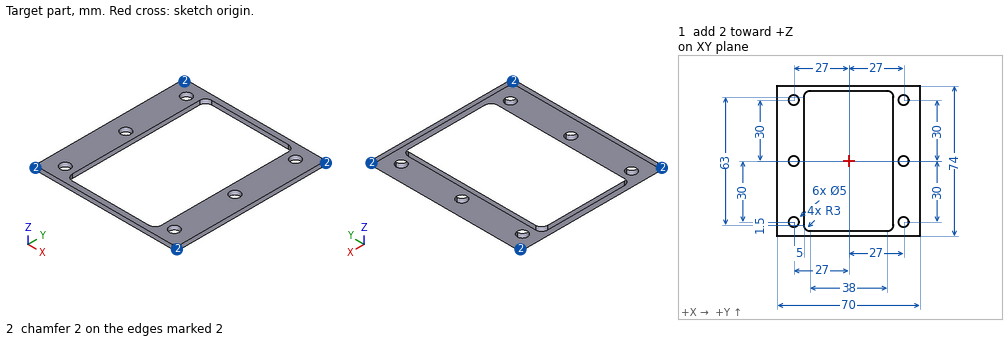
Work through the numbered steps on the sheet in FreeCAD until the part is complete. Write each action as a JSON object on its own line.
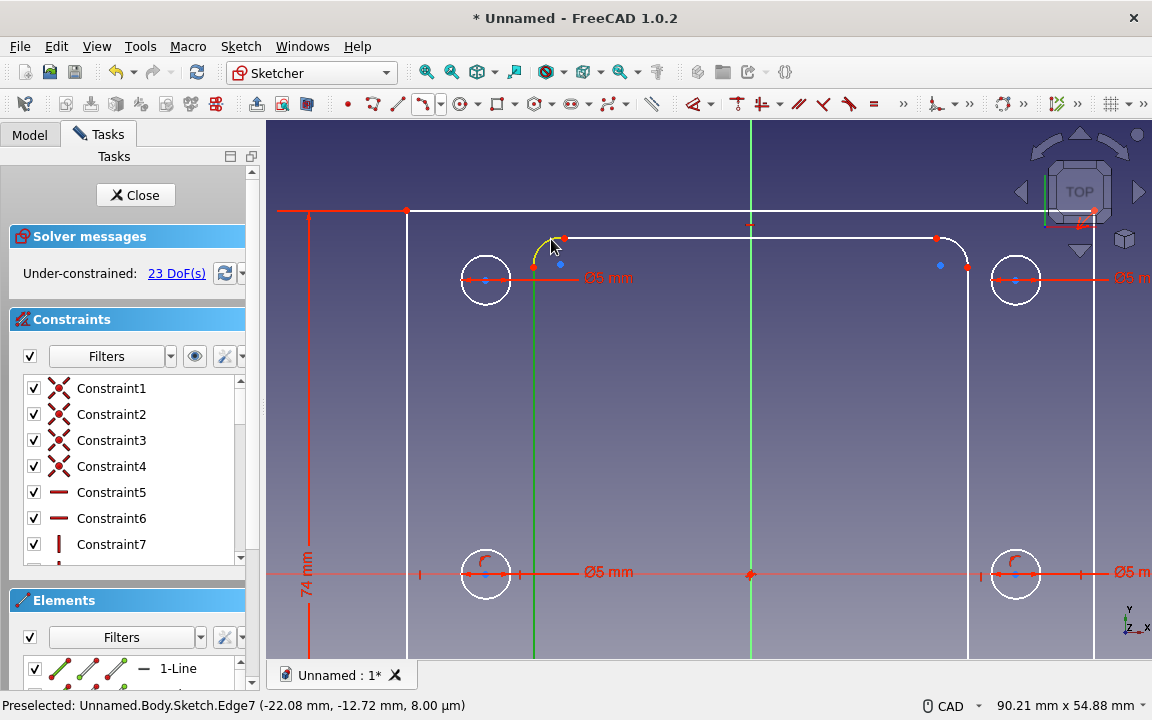
{"action": "left_click", "coordinate": [550, 240]}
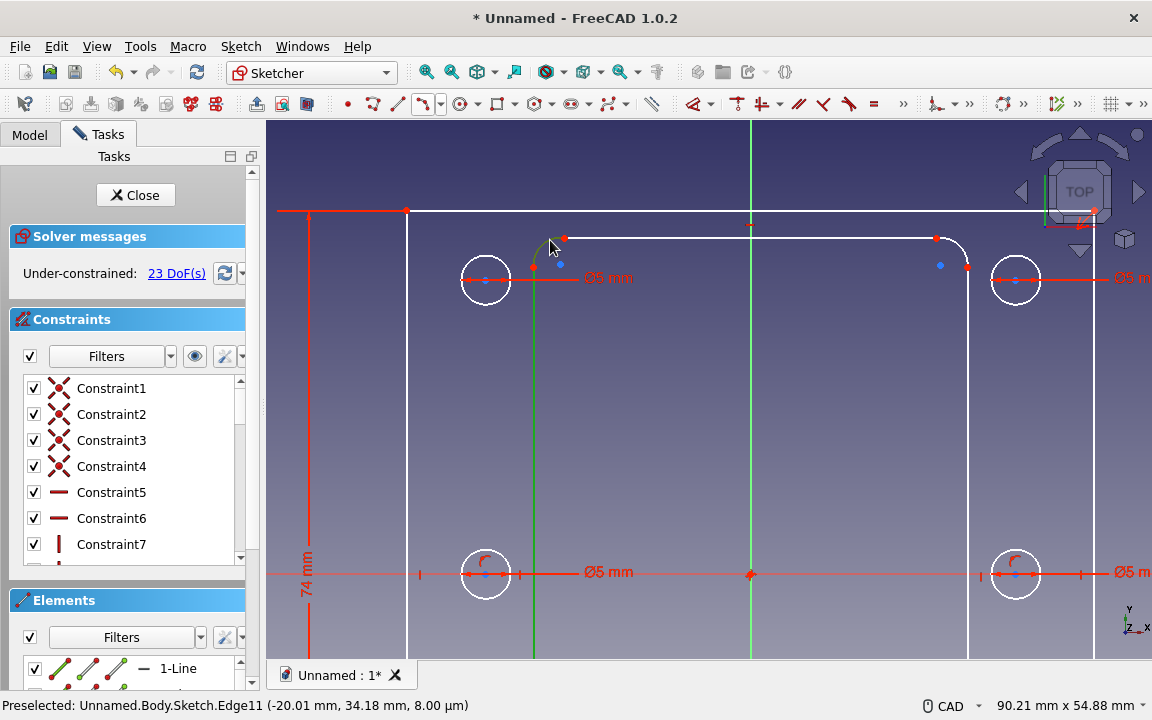
{"action": "left_click", "coordinate": [849, 104]}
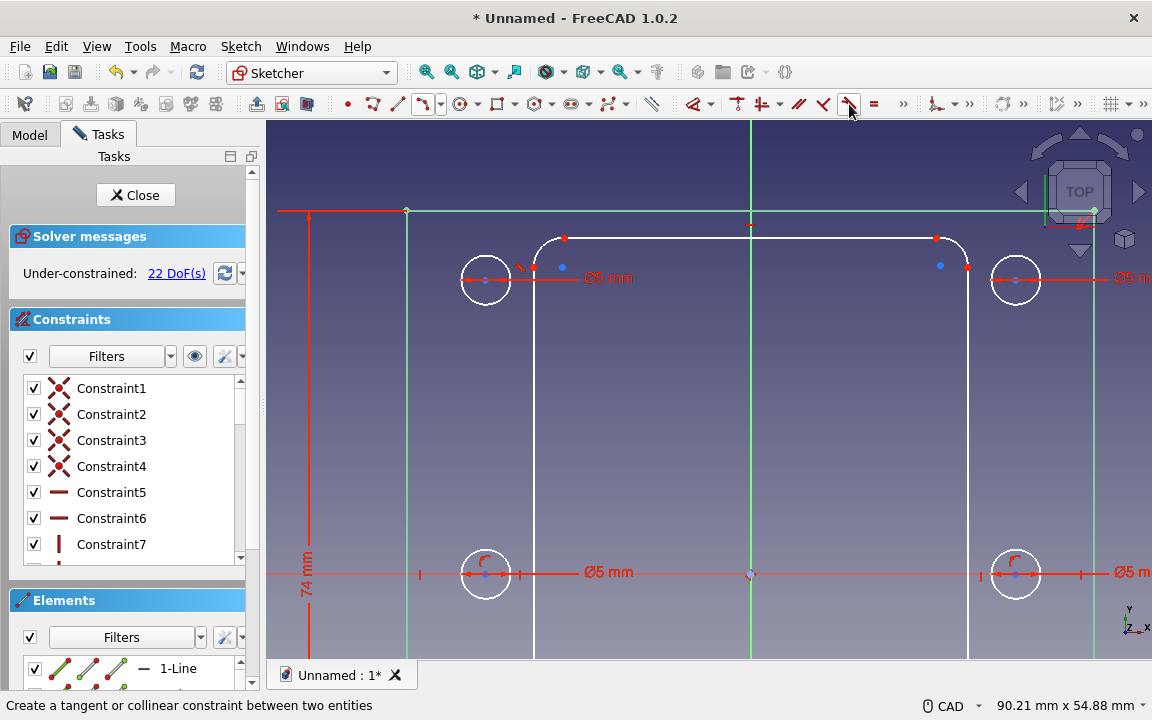
{"action": "left_click", "coordinate": [676, 238]}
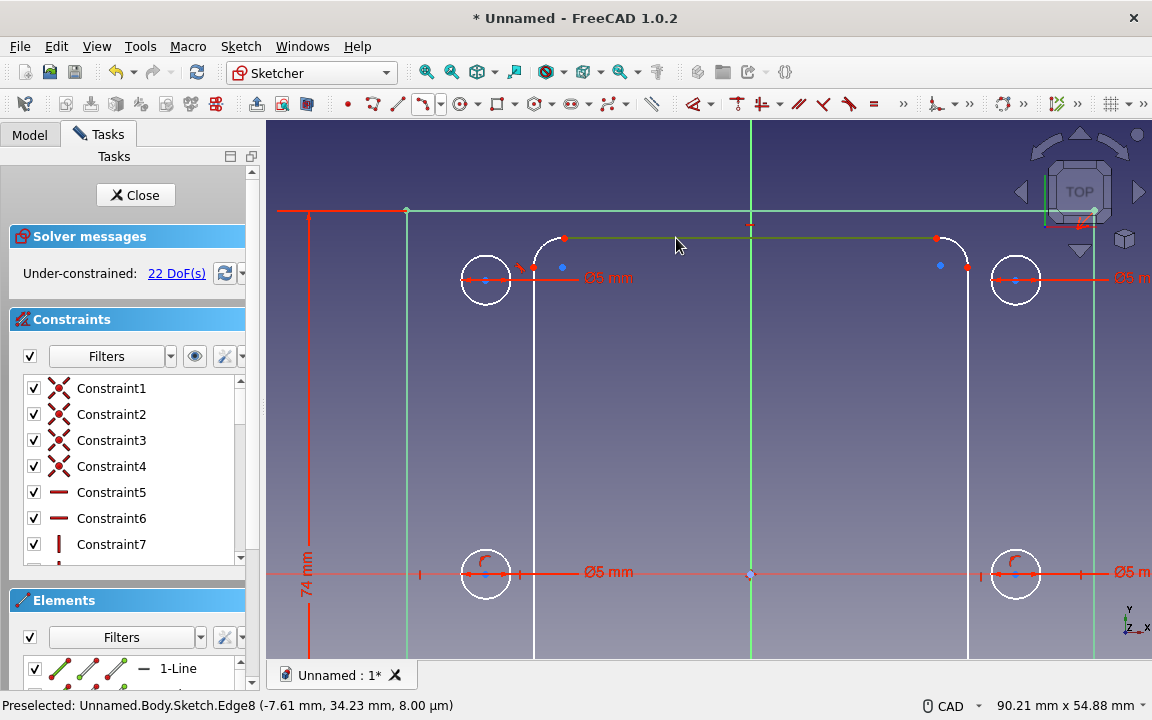
{"action": "left_click", "coordinate": [551, 241]}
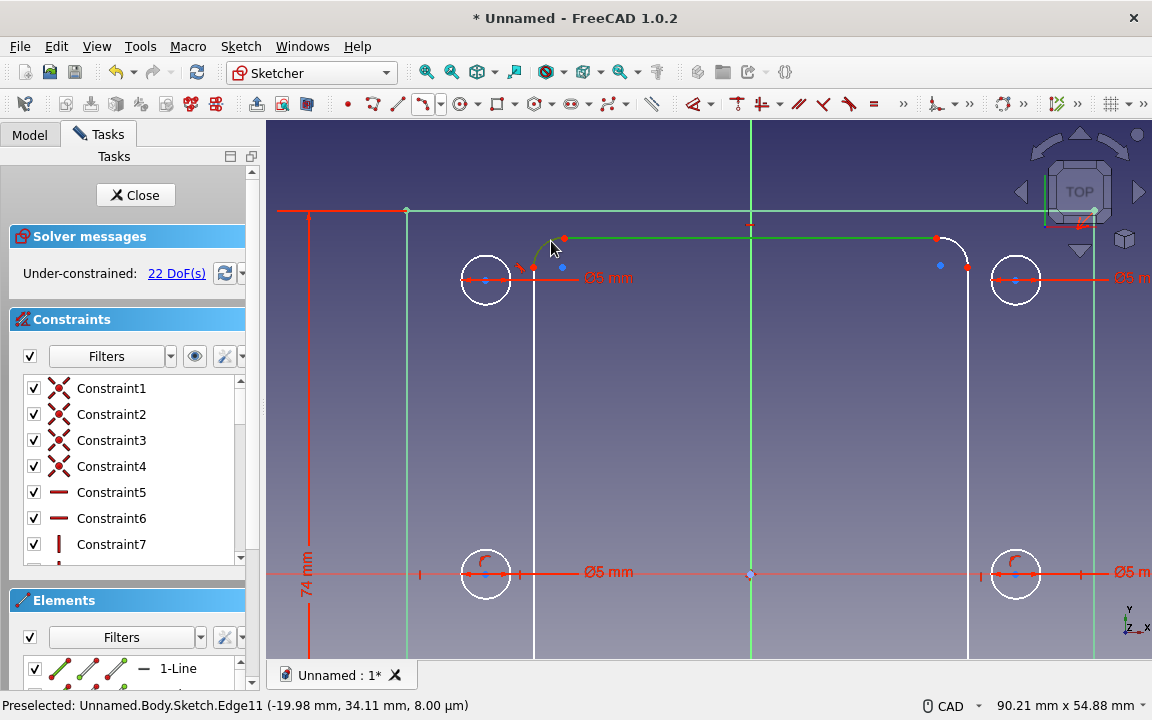
{"action": "left_click", "coordinate": [849, 104]}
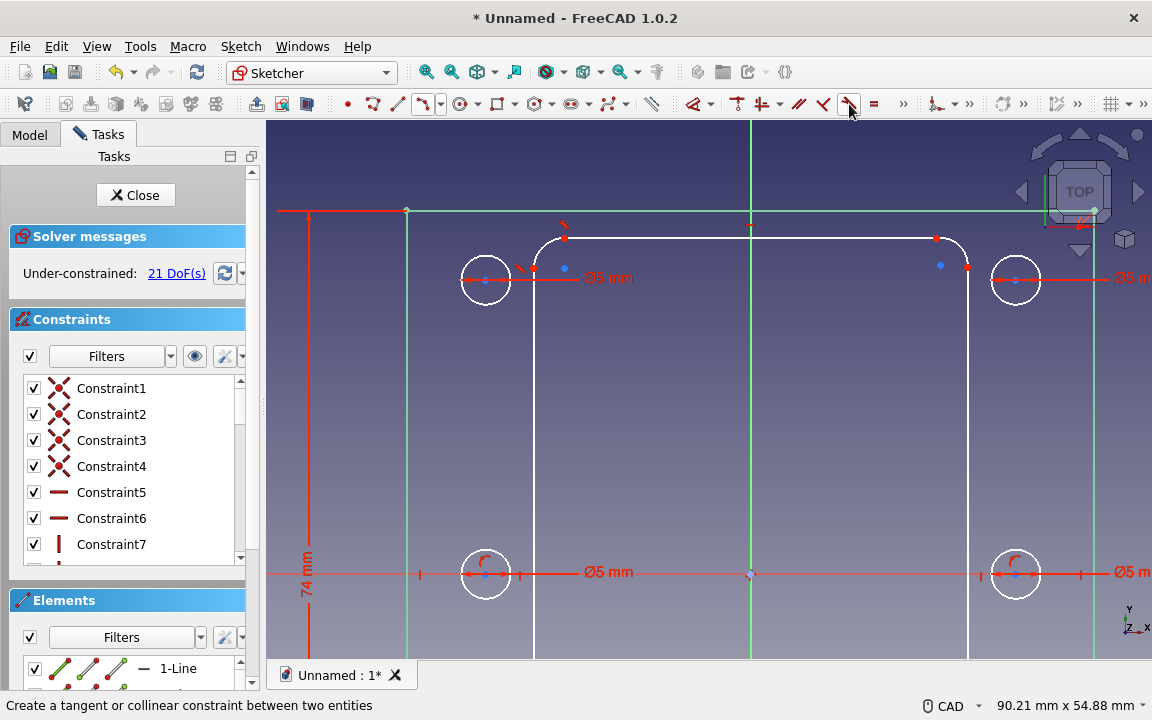
{"action": "left_click", "coordinate": [676, 238]}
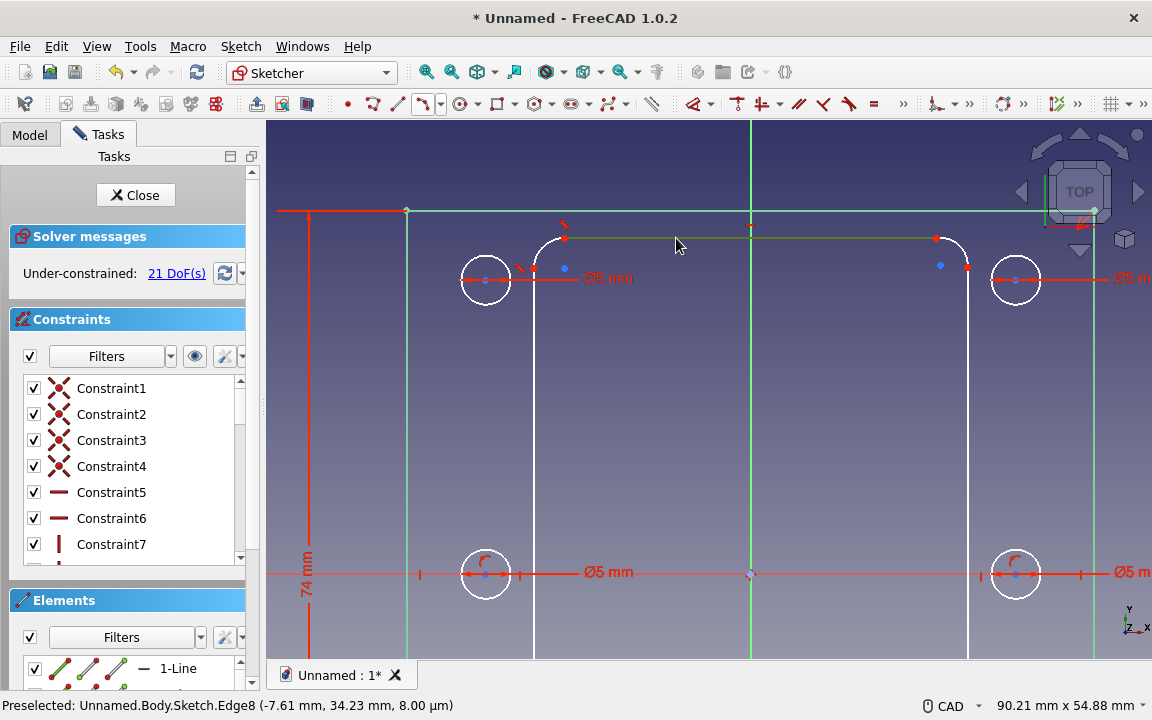
{"action": "left_click", "coordinate": [965, 253]}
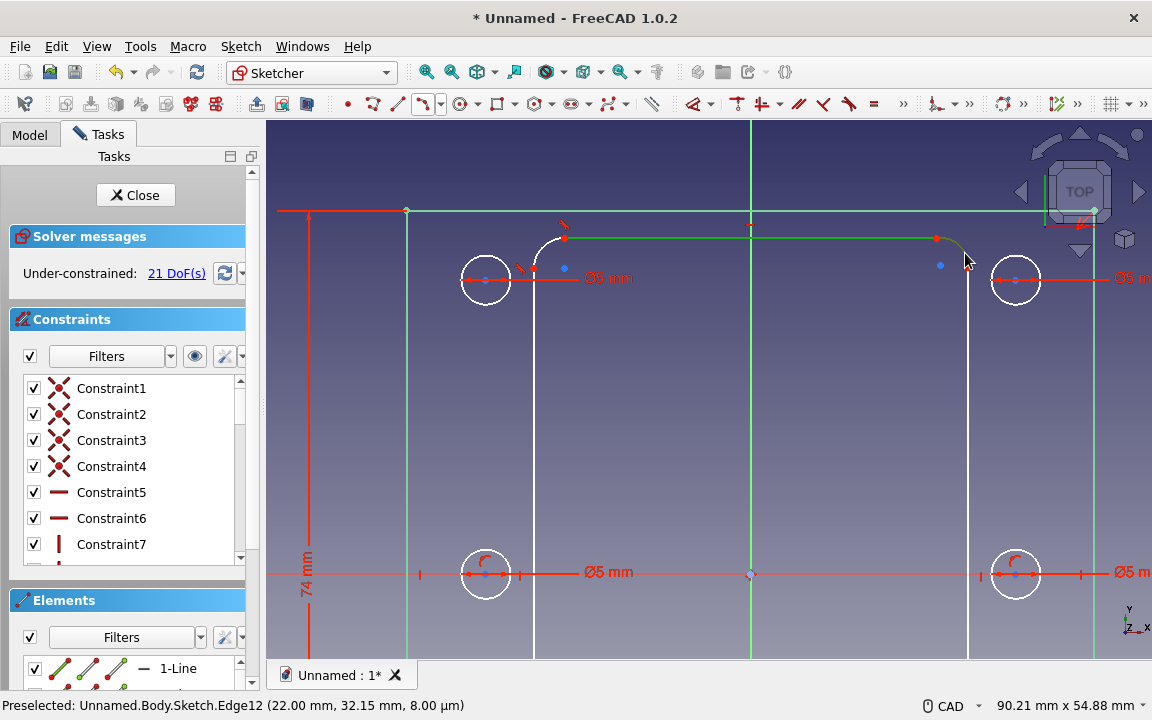
{"action": "left_click", "coordinate": [849, 104]}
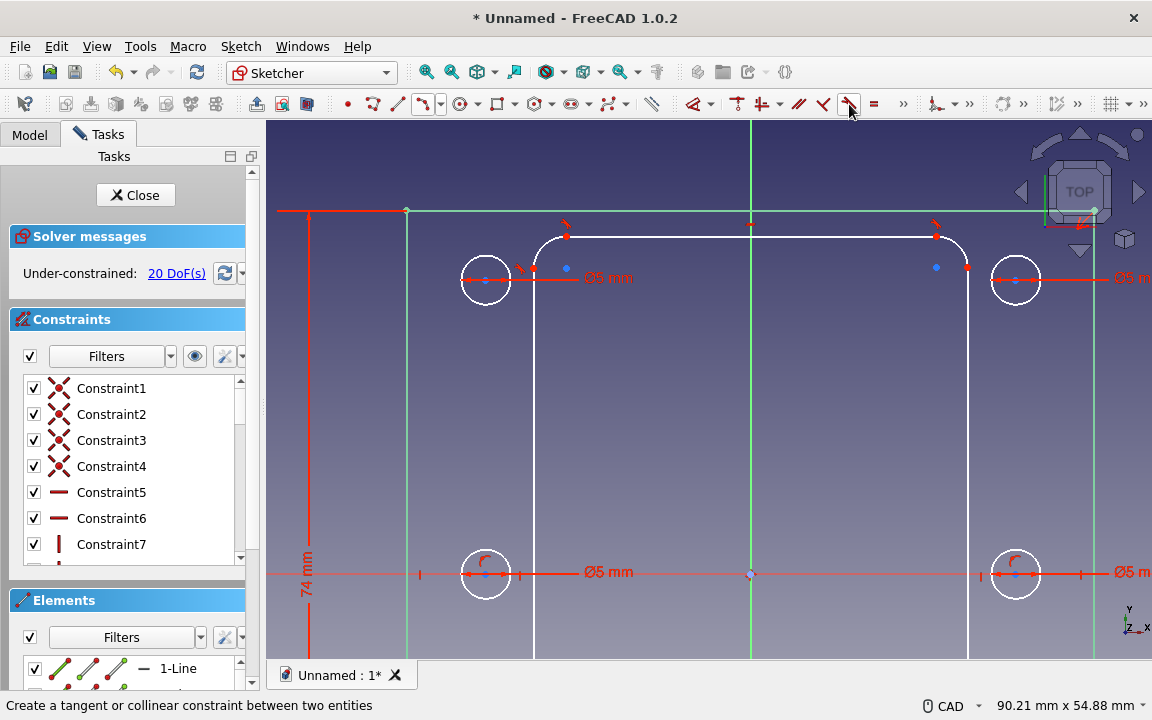
{"action": "left_click", "coordinate": [968, 453]}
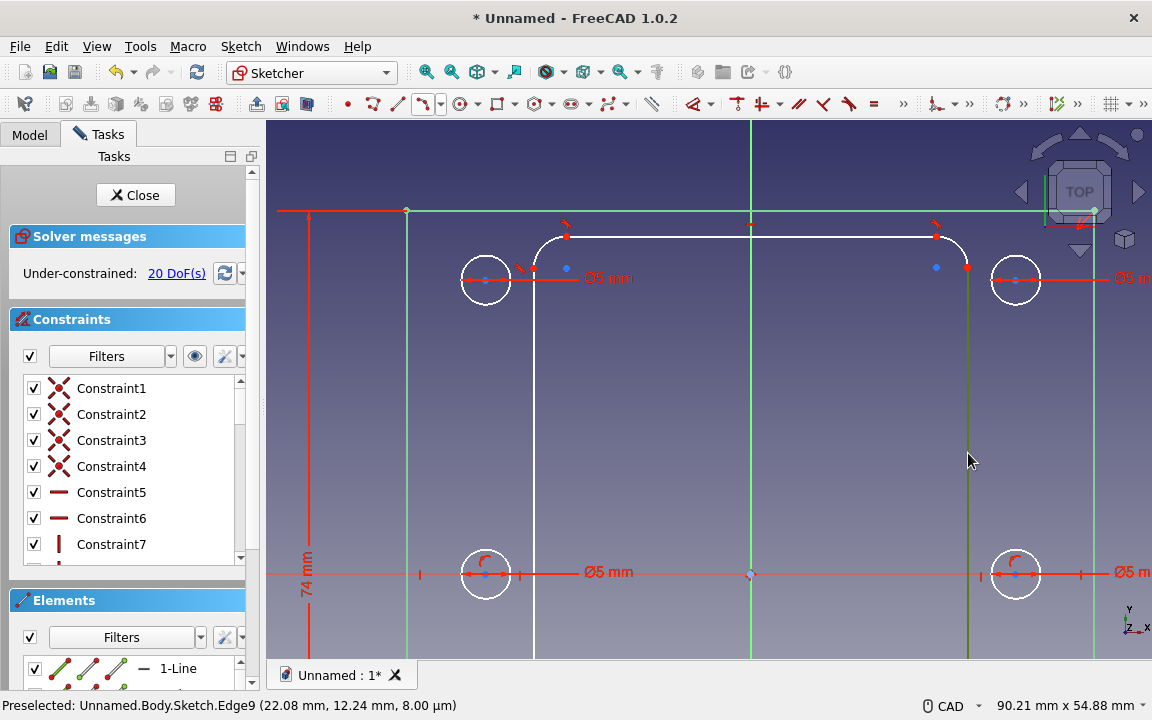
{"action": "left_click", "coordinate": [964, 253]}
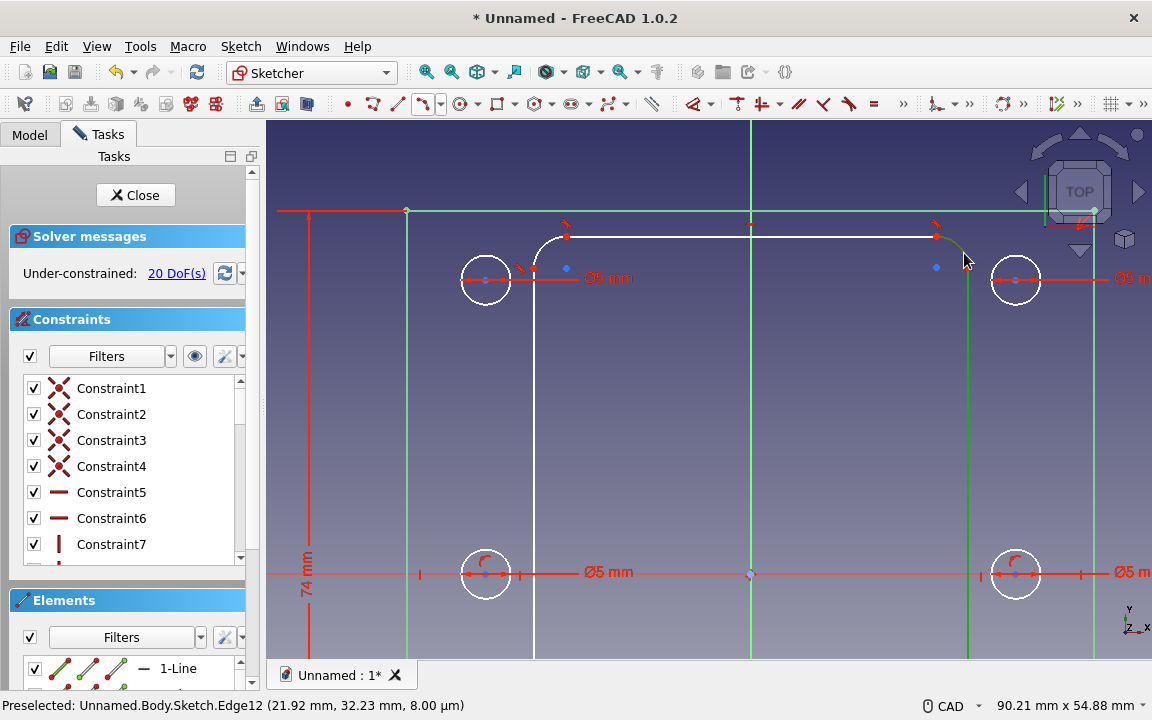
{"action": "left_click", "coordinate": [849, 104]}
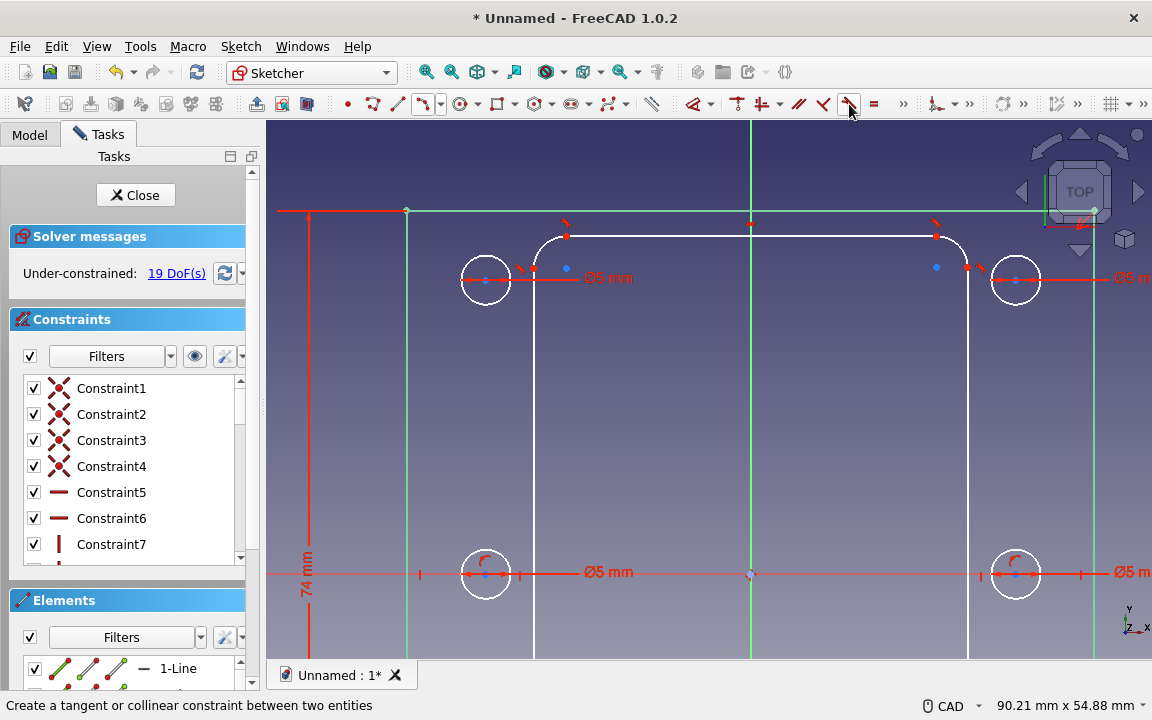
{"action": "left_click", "coordinate": [968, 453]}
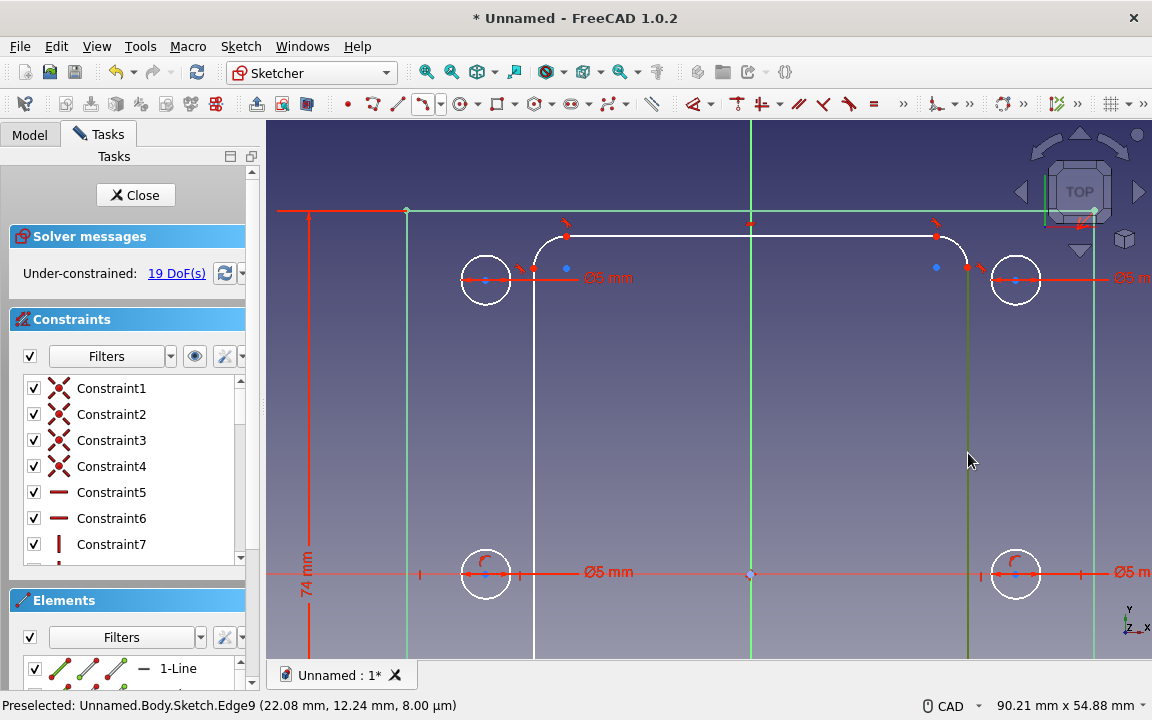
{"action": "scroll", "coordinate": [551, 239], "scroll_direction": "down", "scroll_amount": 4}